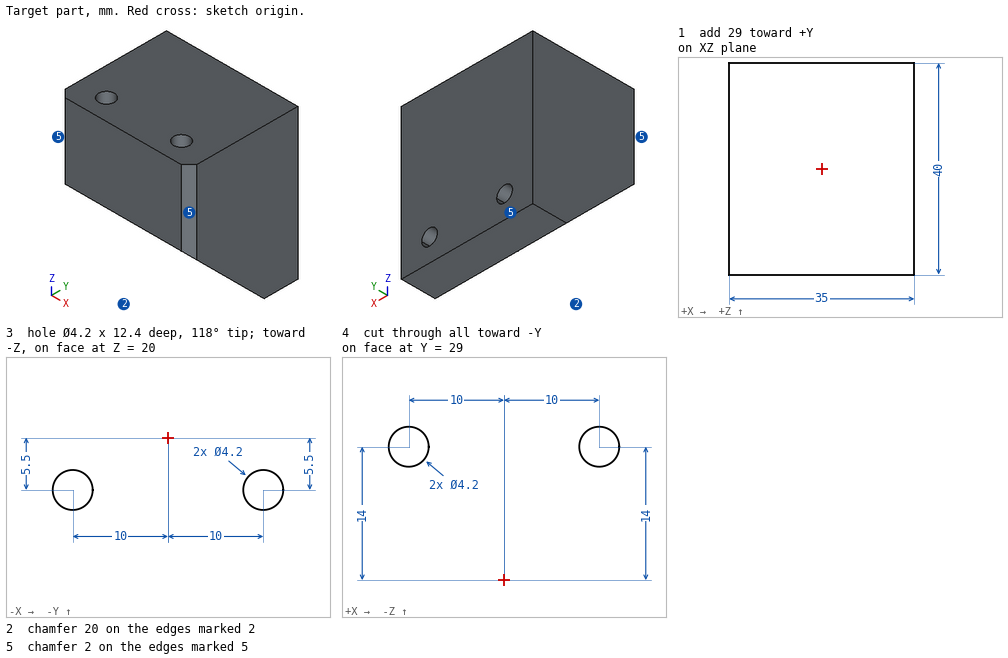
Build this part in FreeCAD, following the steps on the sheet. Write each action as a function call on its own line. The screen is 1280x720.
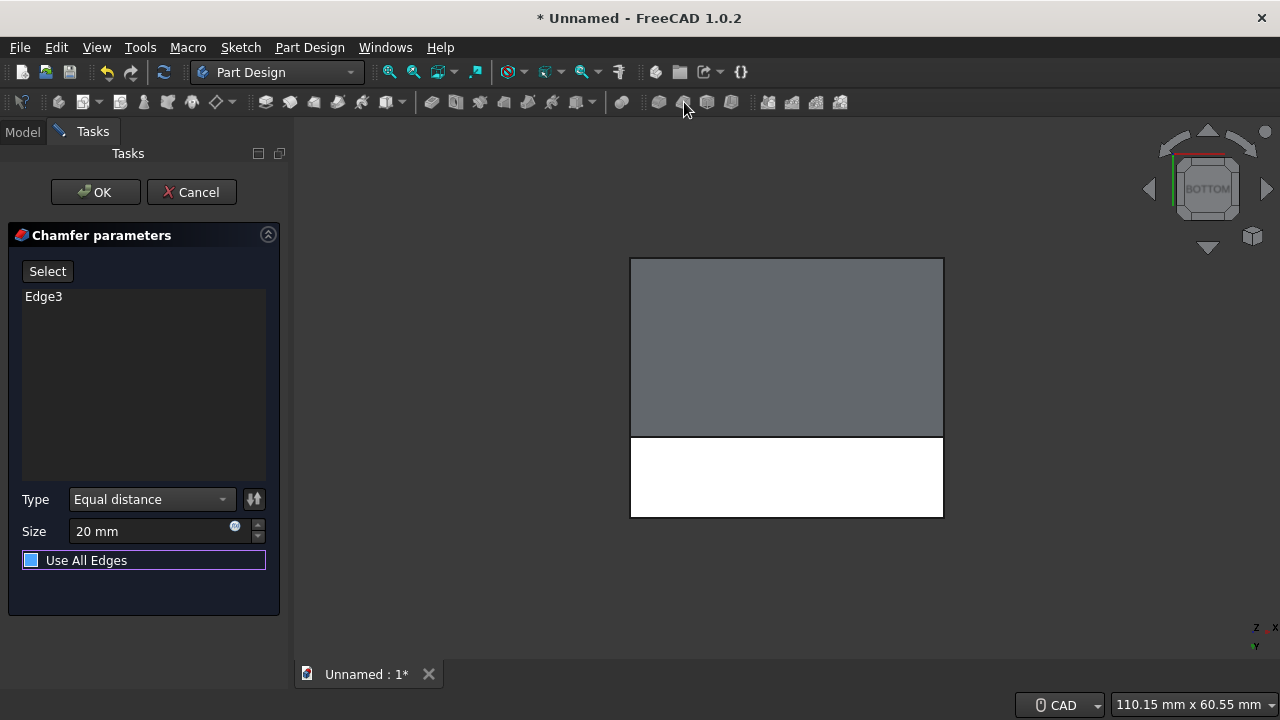
click(96, 192)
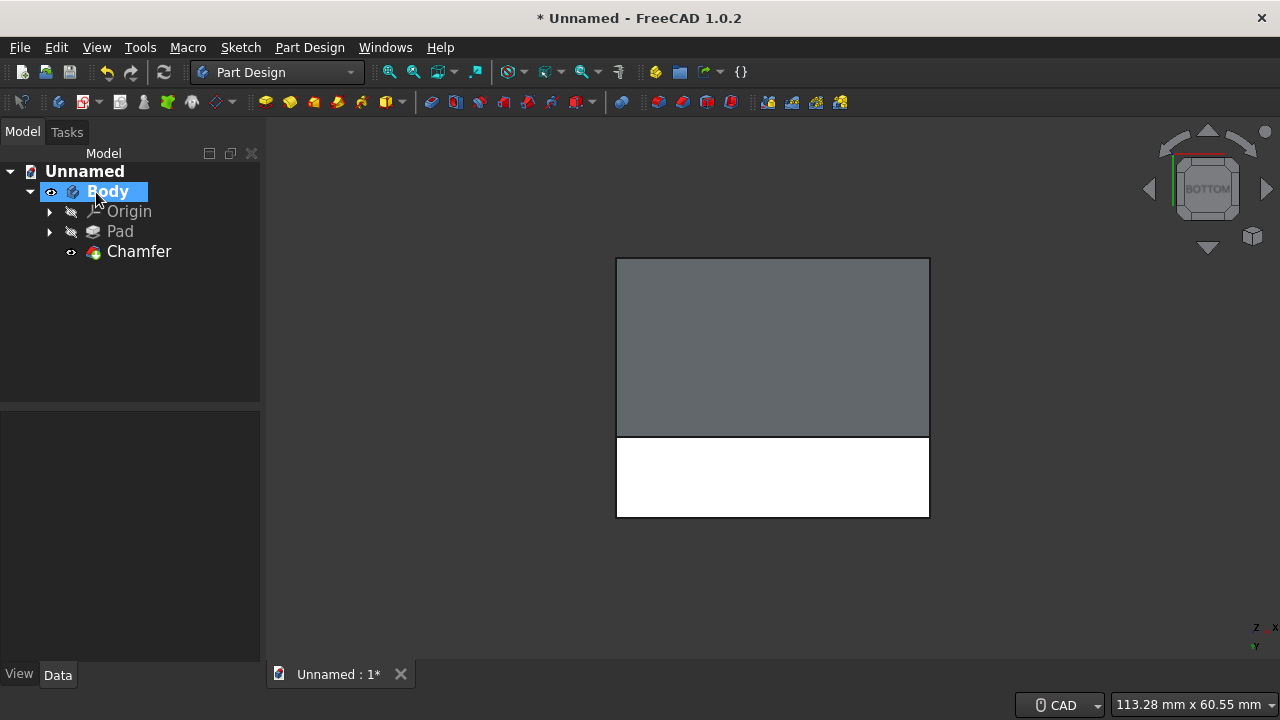
key(0)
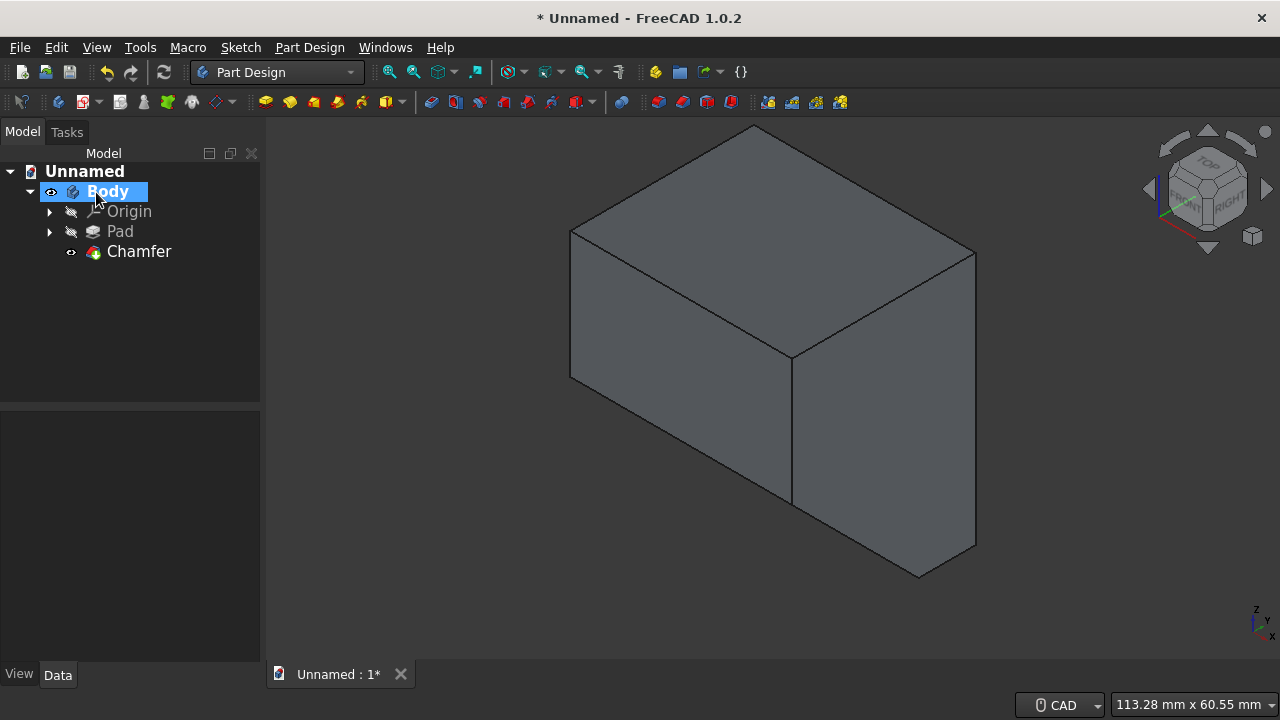
click(773, 241)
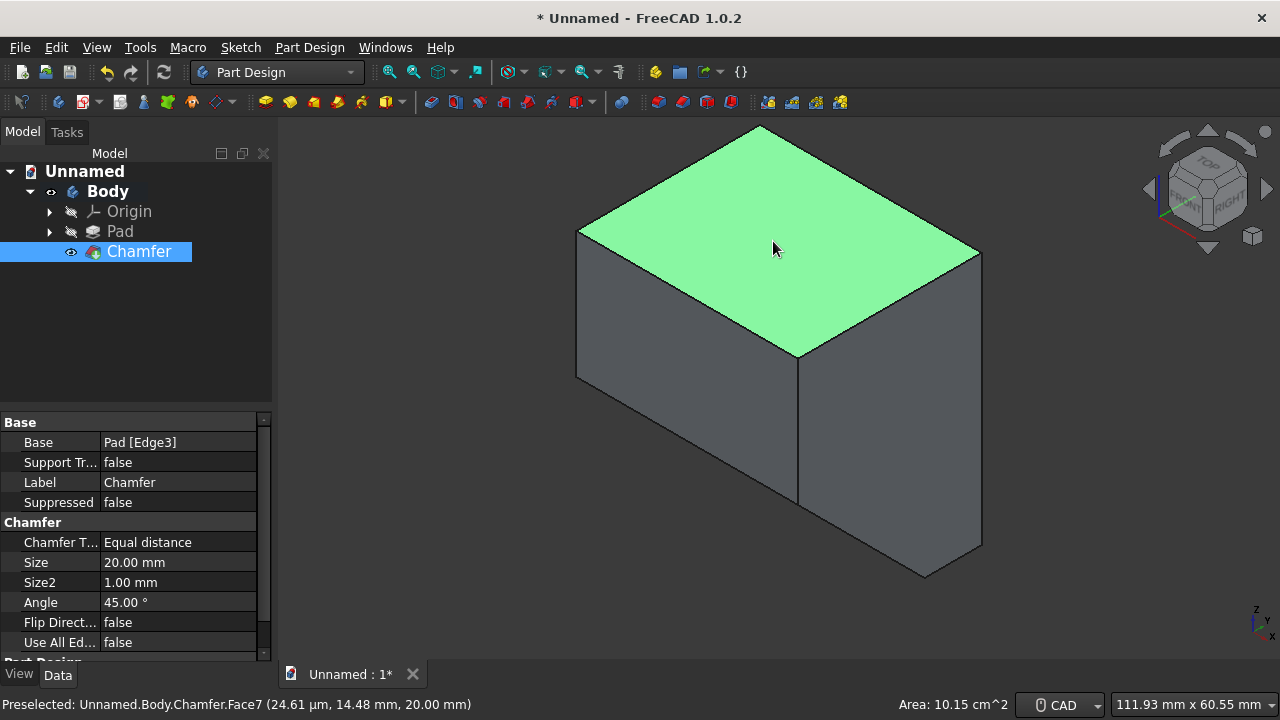
click(84, 102)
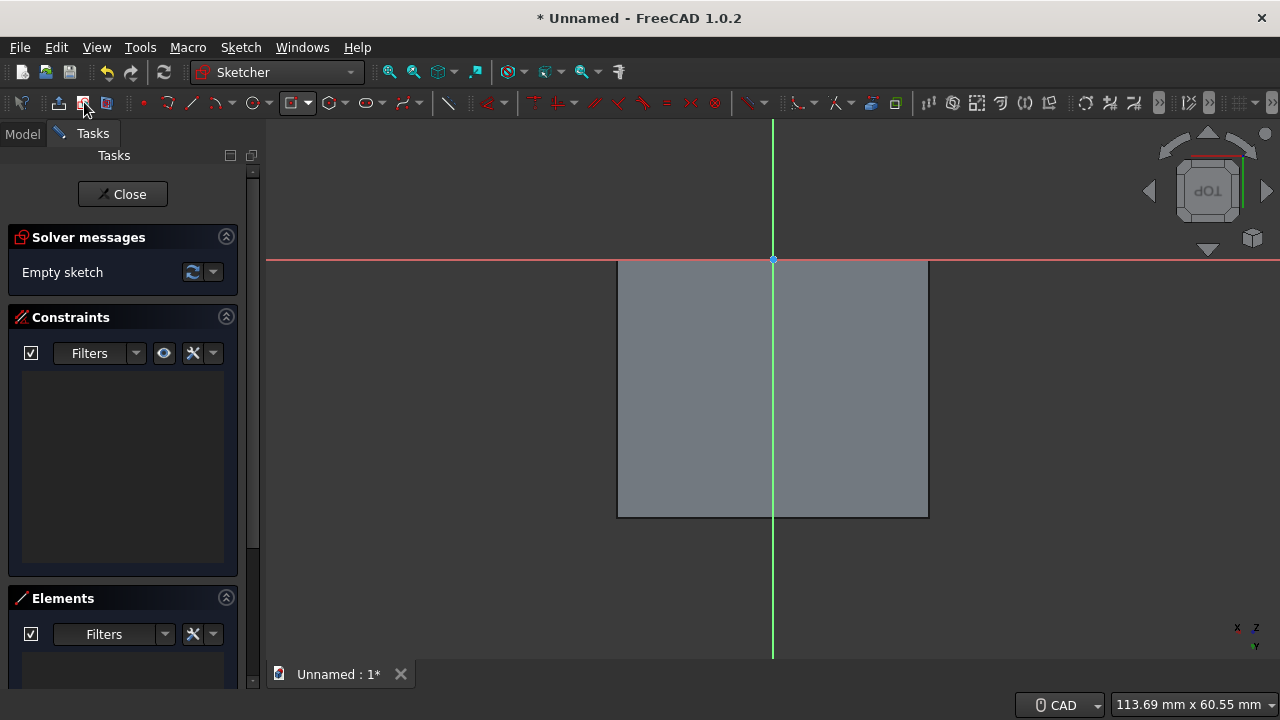
scroll(813, 238, up, 5)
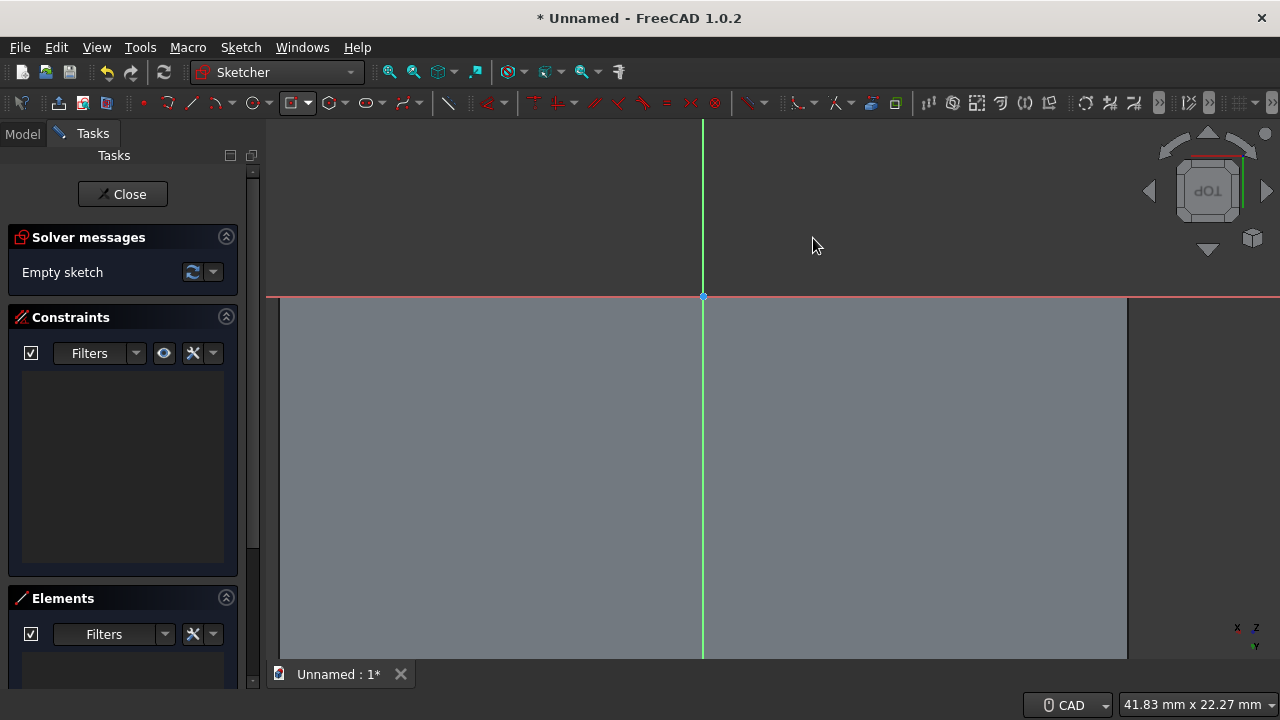
key(g)
key(c)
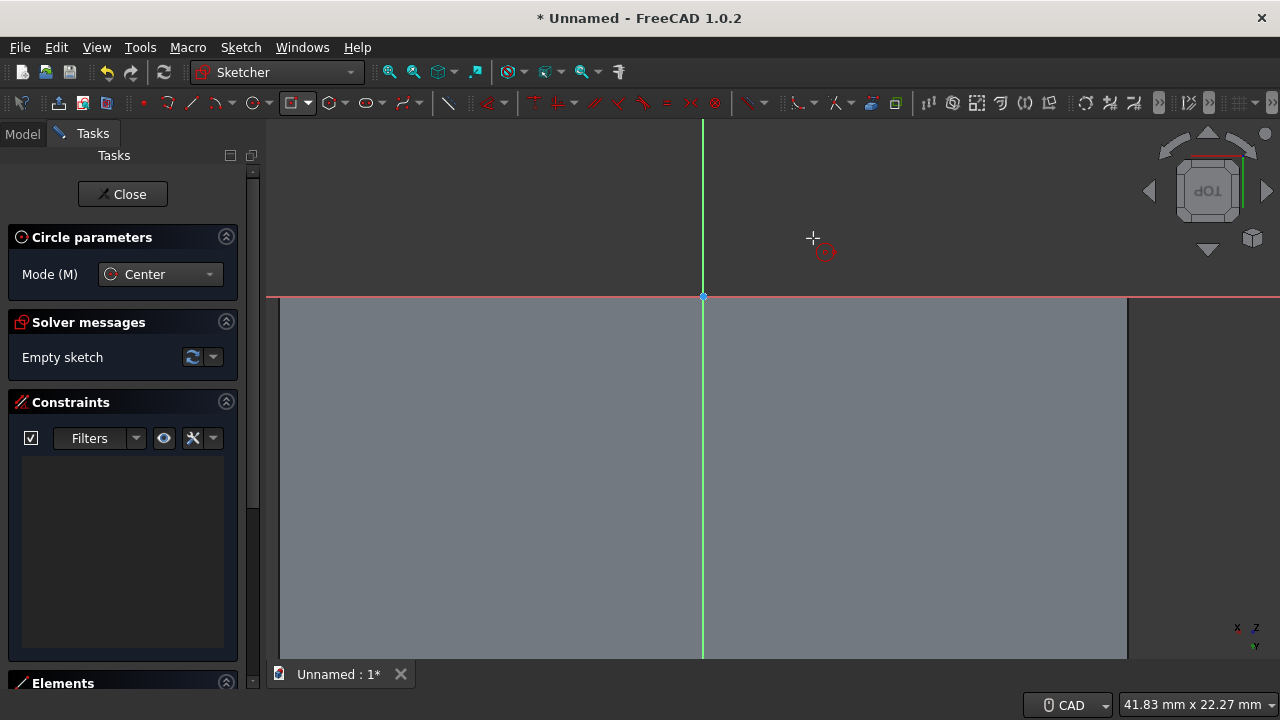
click(946, 430)
move(982, 394)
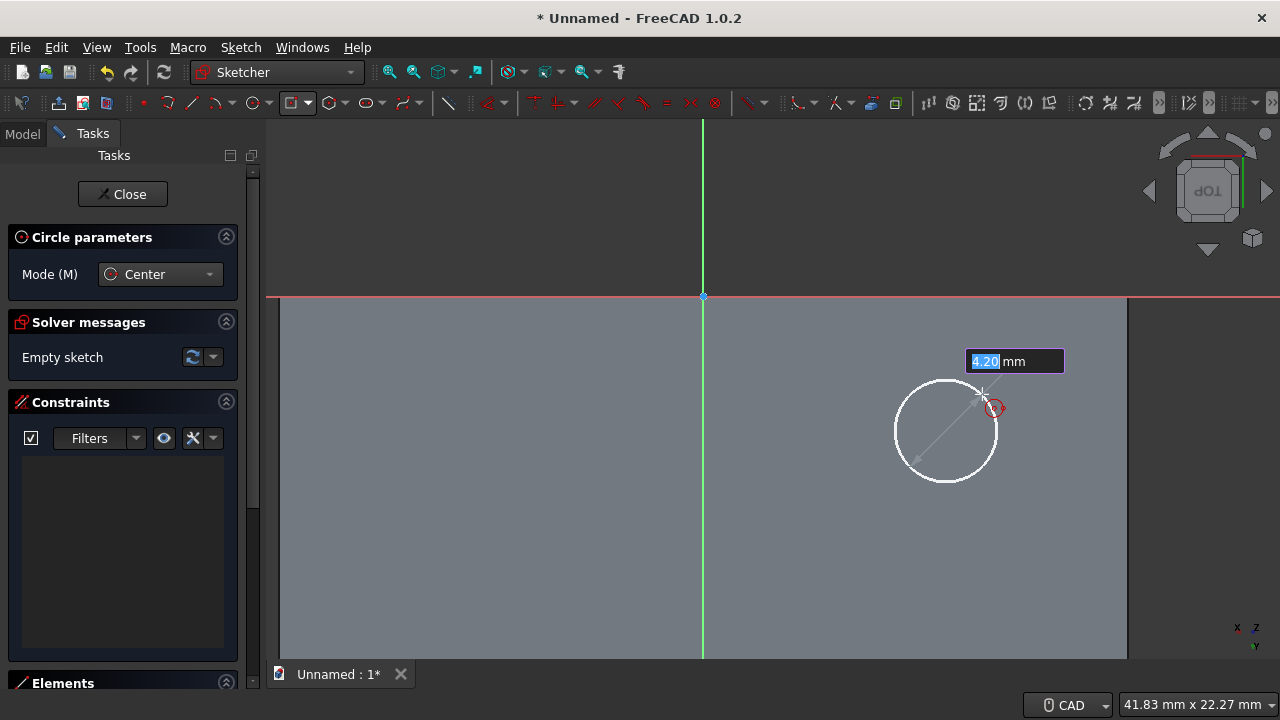
text(4.2)
key(Return)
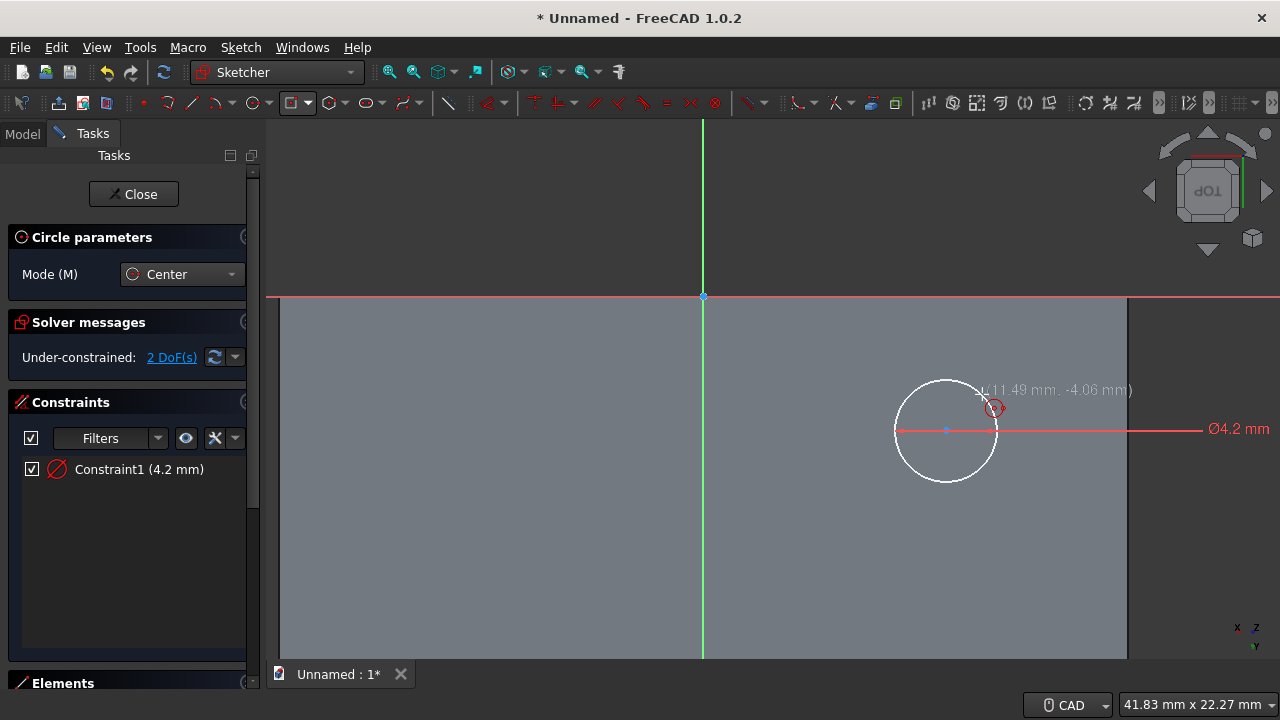
click(461, 430)
move(497, 394)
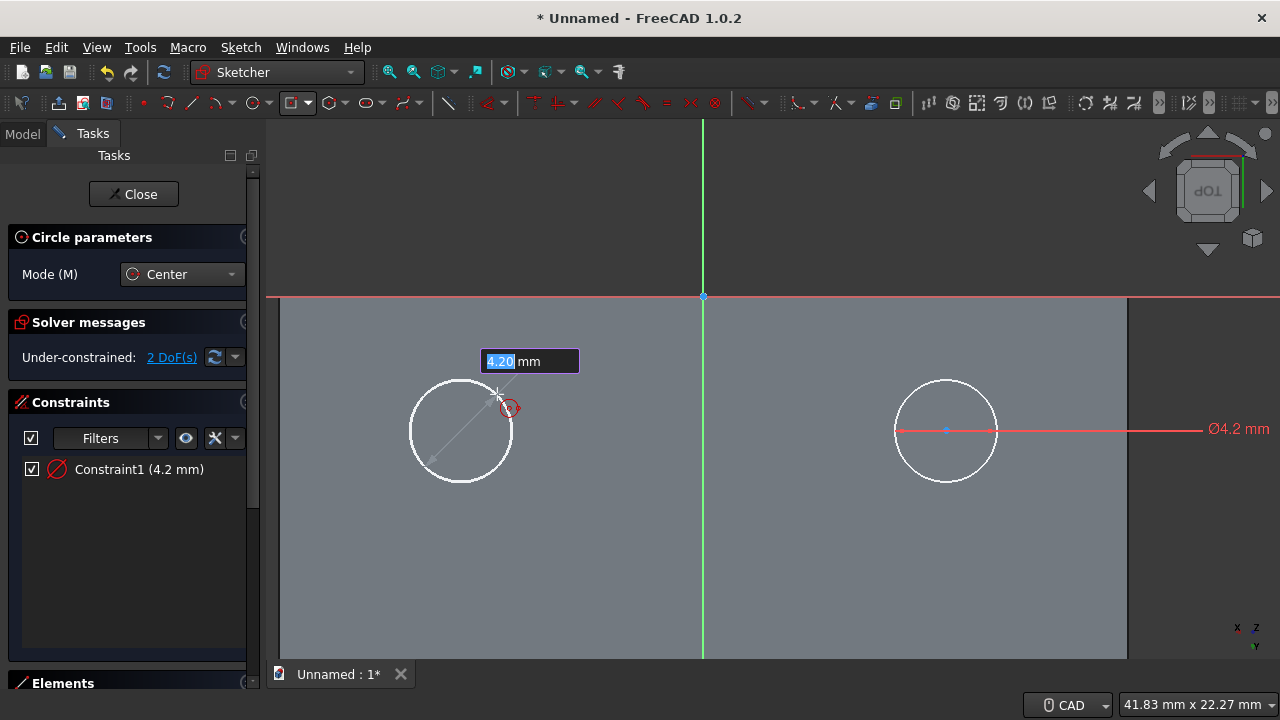
text(4.2)
key(Return)
key(Escape)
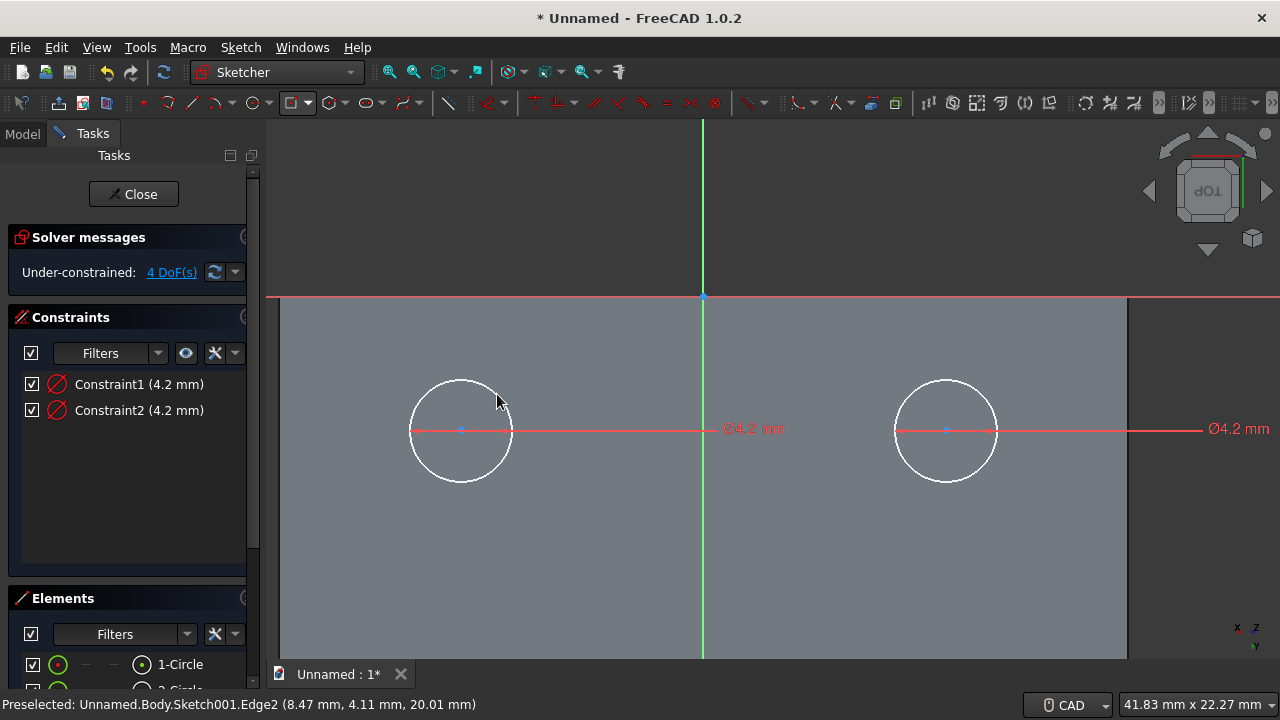
key(d)